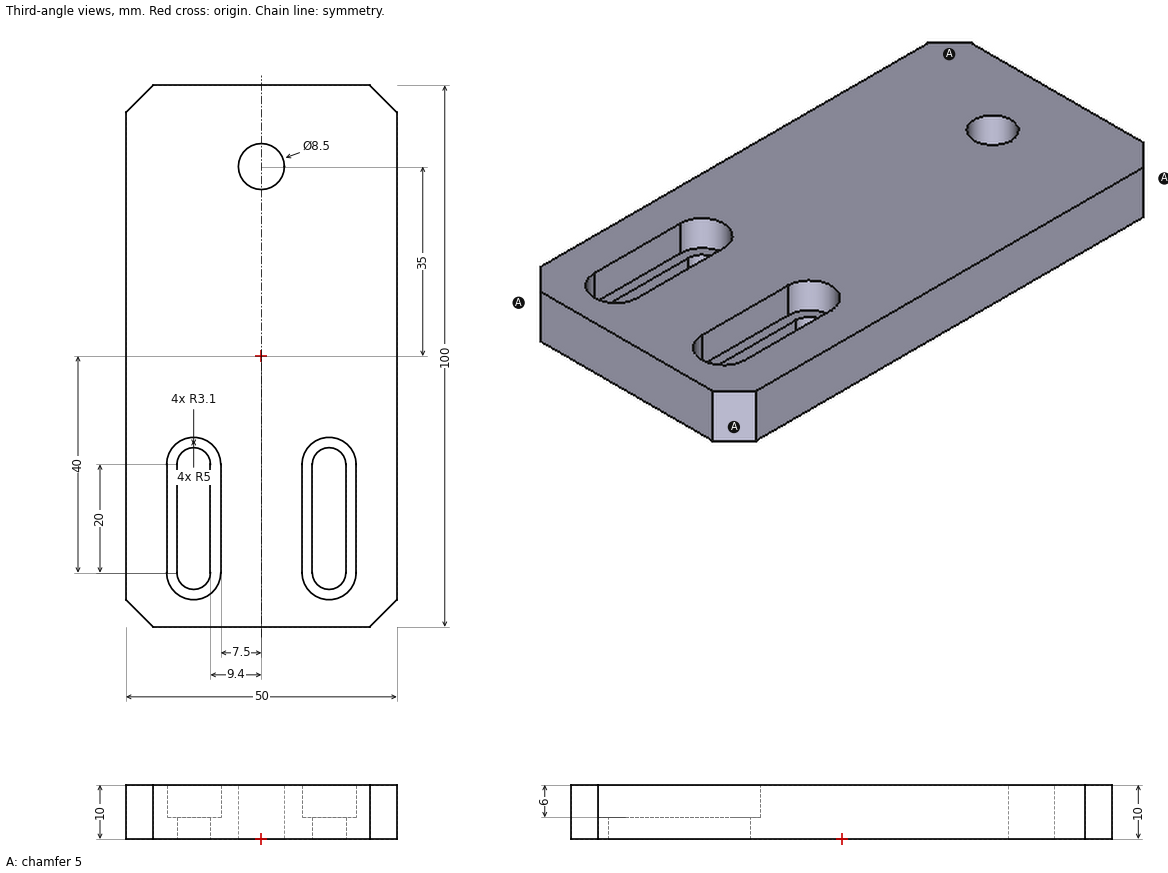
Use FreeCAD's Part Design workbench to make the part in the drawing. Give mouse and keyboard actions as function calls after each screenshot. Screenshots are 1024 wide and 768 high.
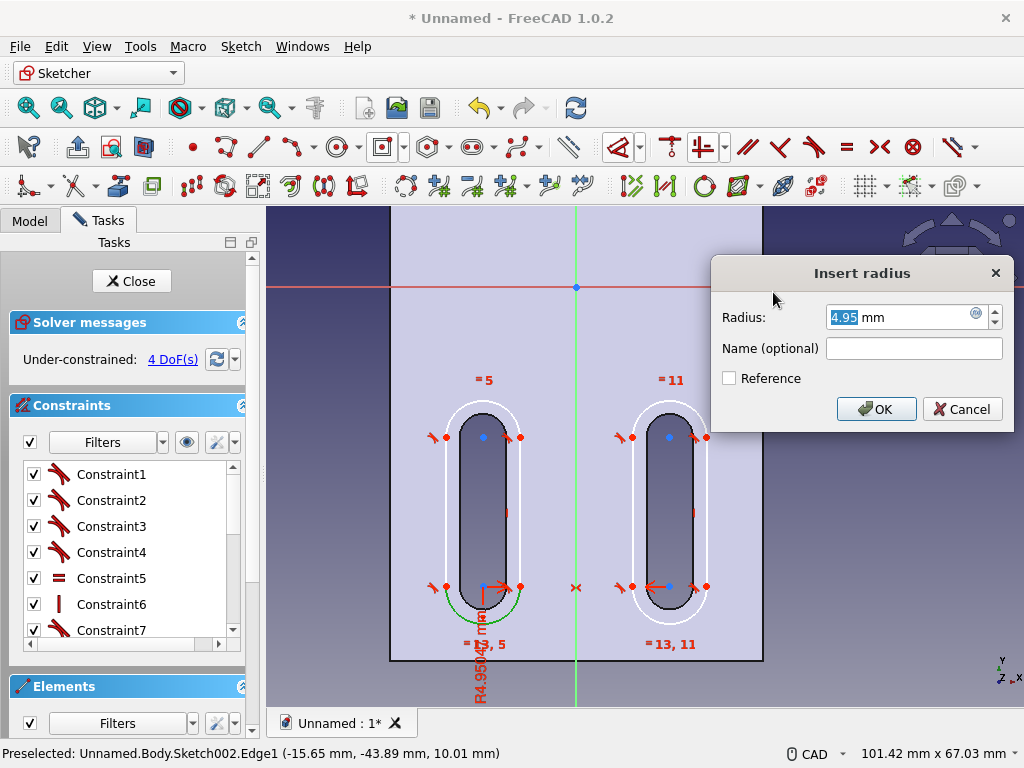
text(5)
key(Return)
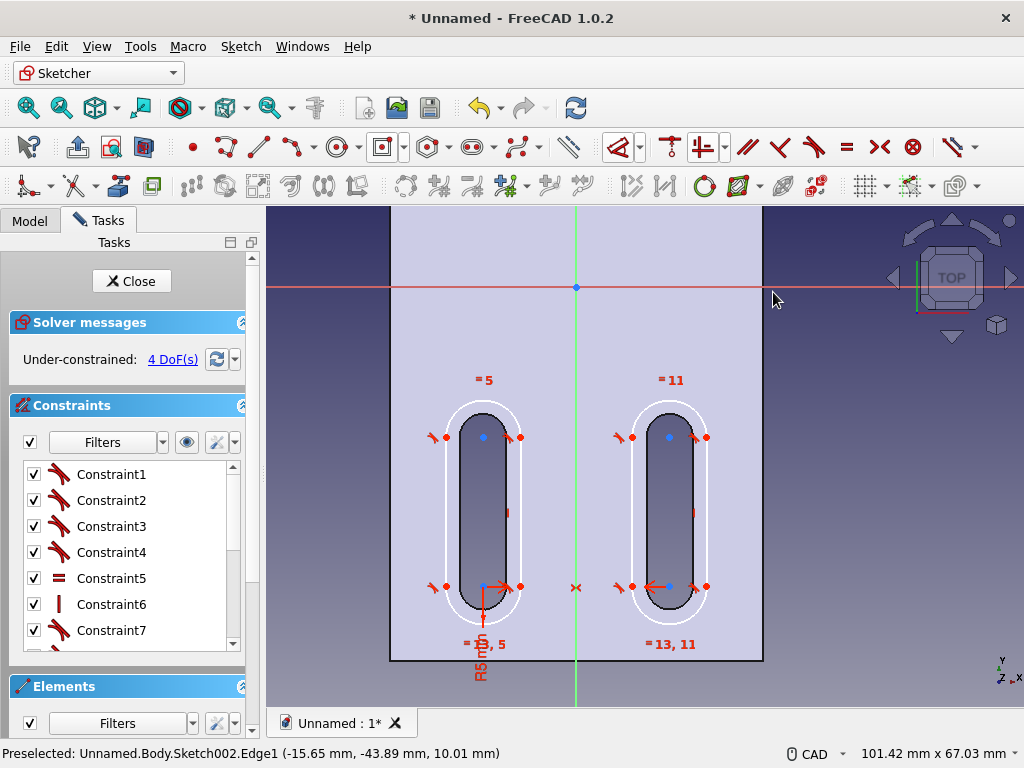
click(446, 542)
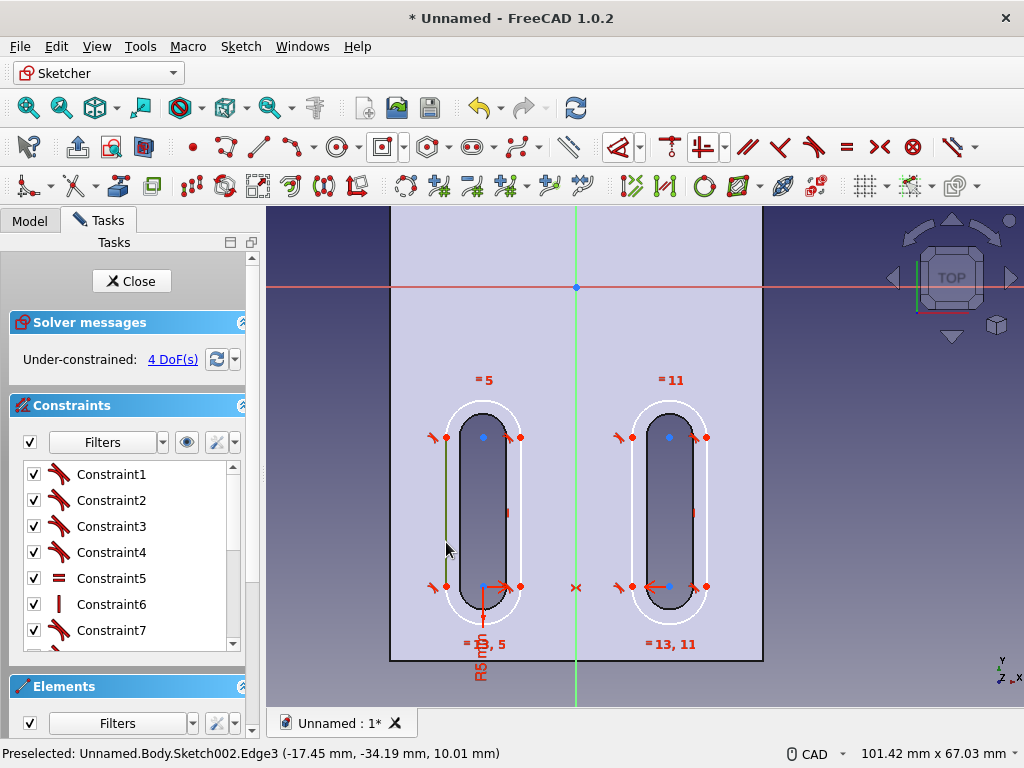
key(i)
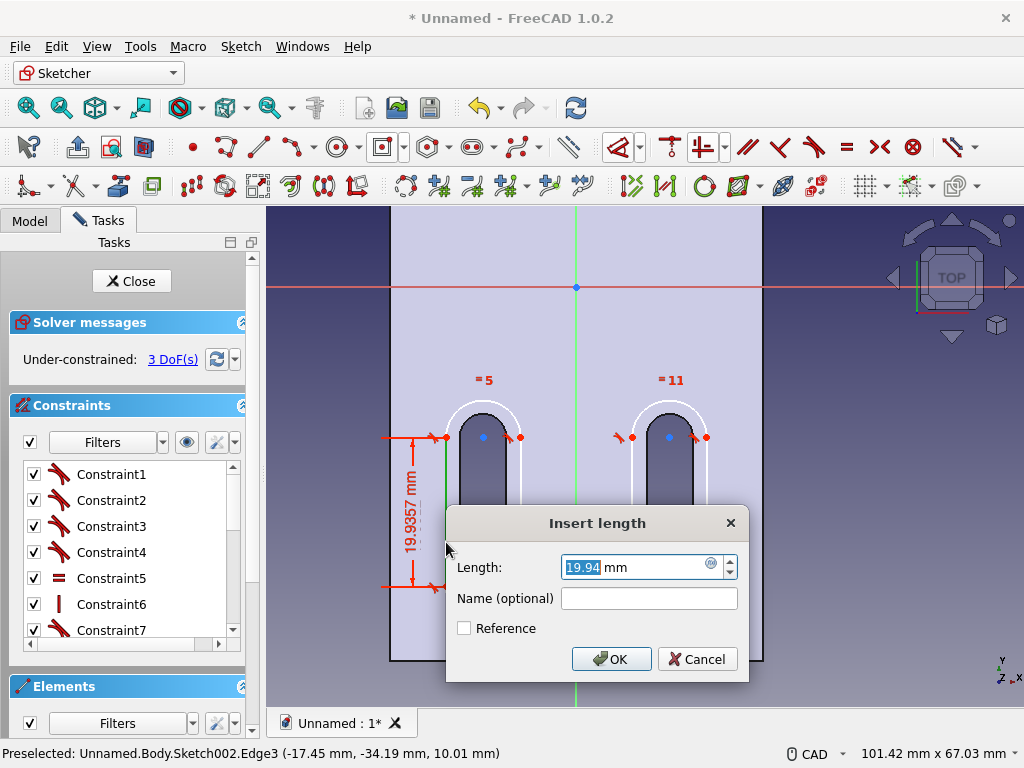
text(20)
key(Return)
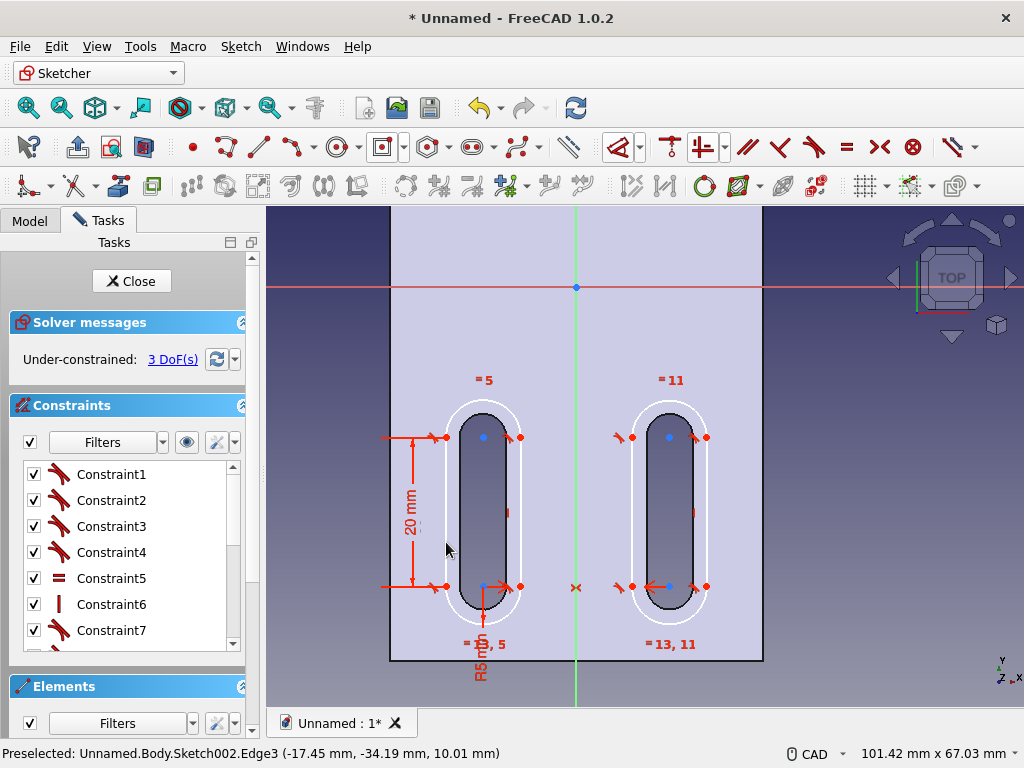
click(632, 542)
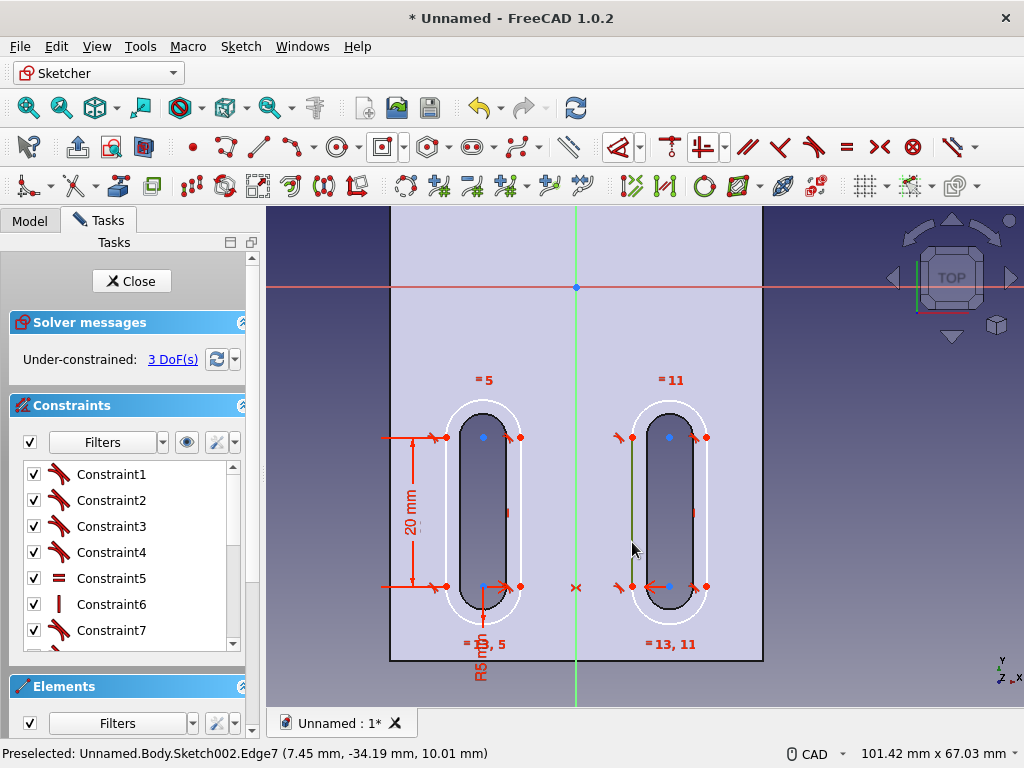
click(640, 148)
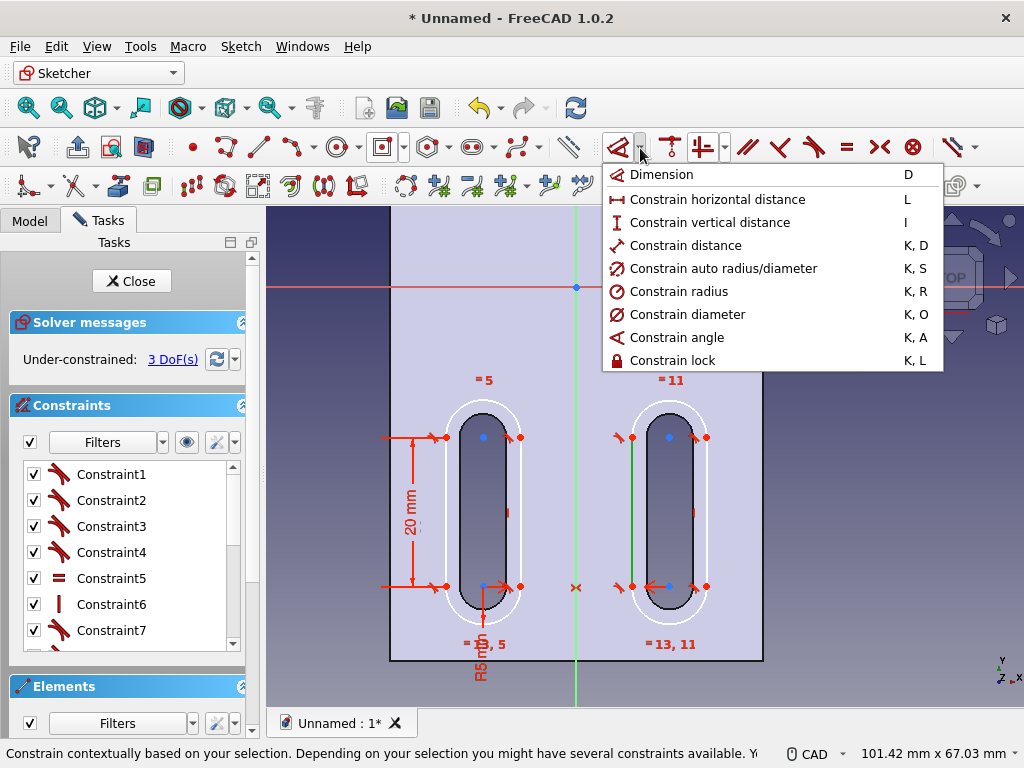
click(773, 222)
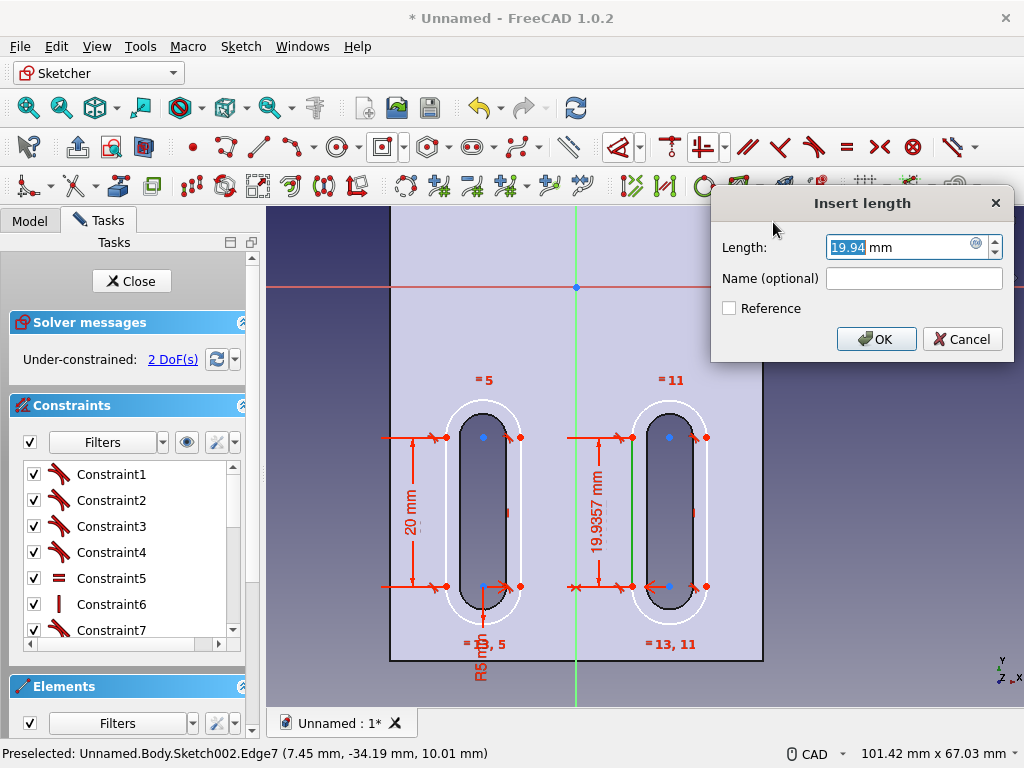
text(20)
key(Return)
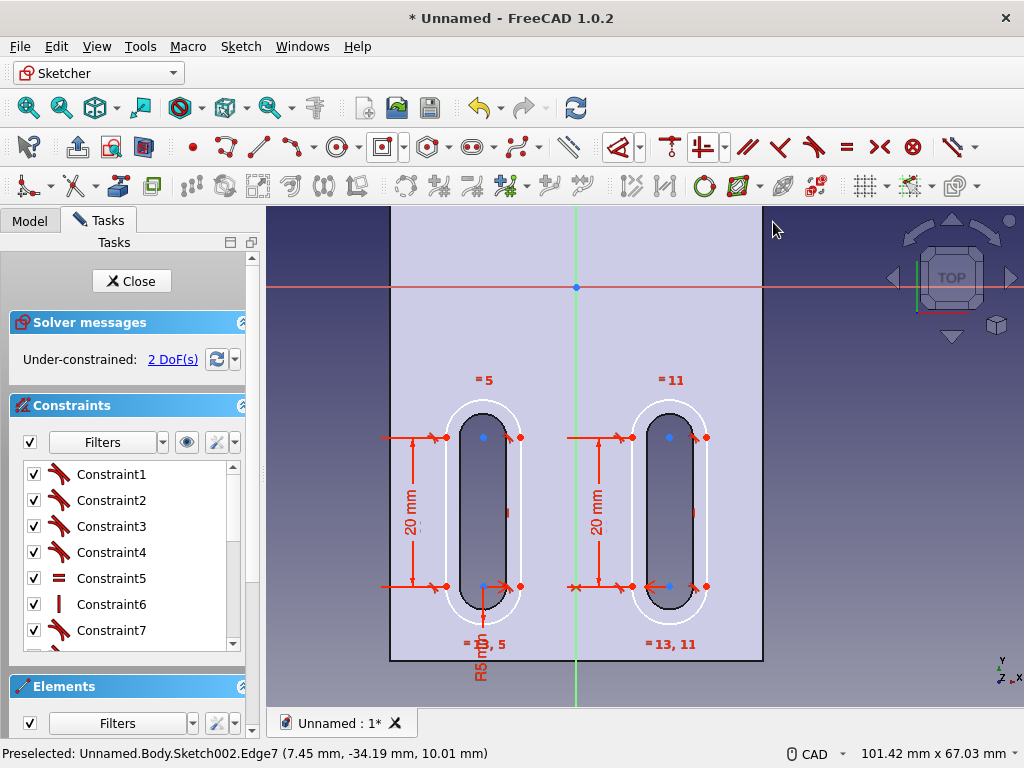
click(446, 587)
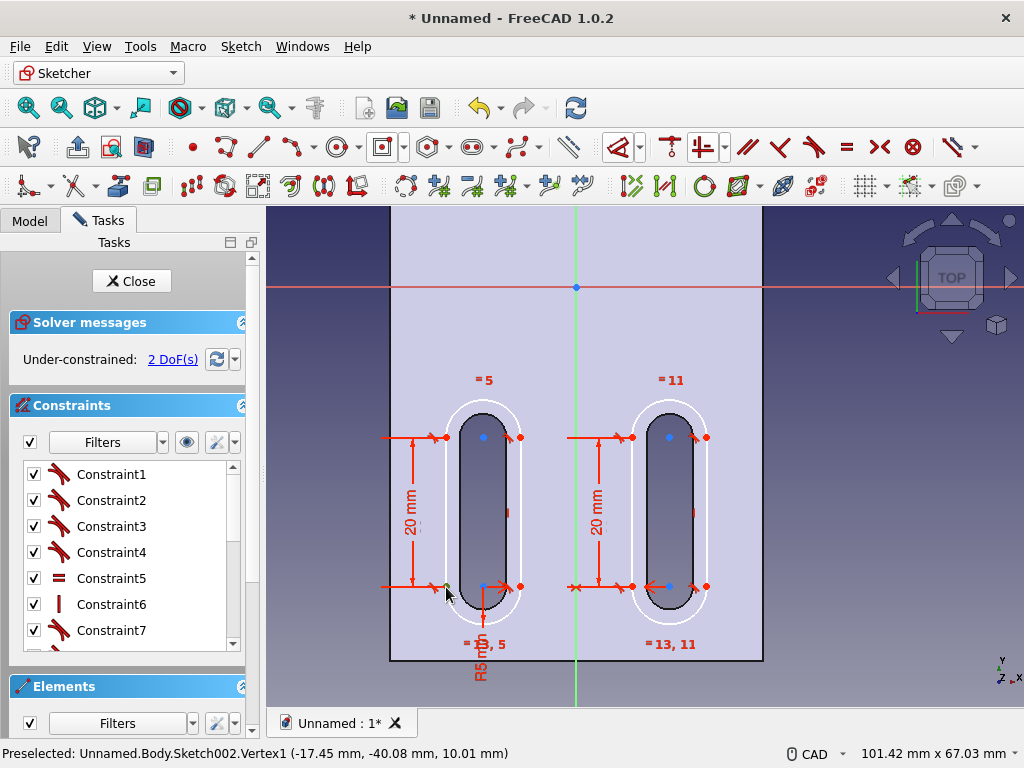
key(i)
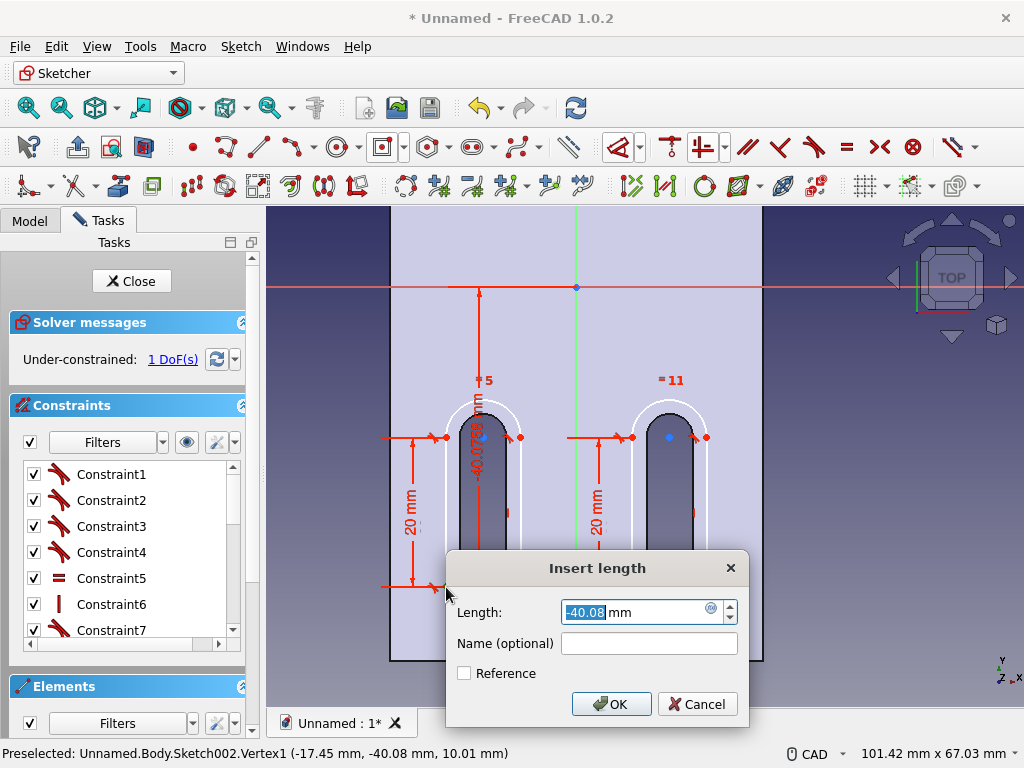
text(-40)
key(Return)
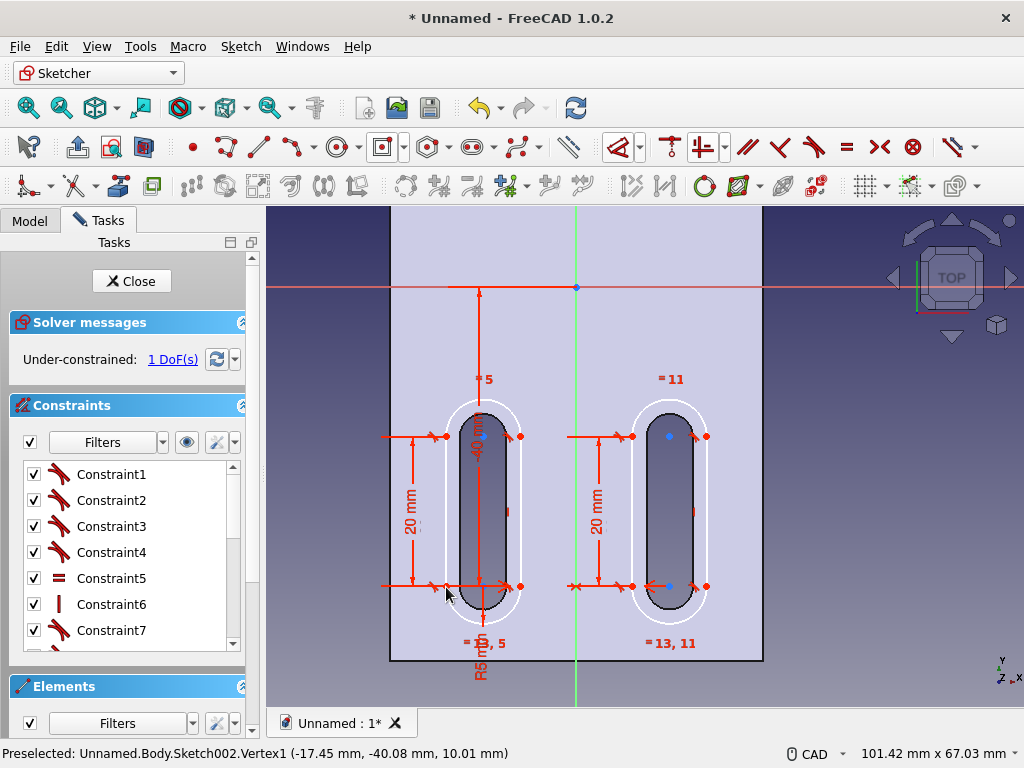
click(521, 586)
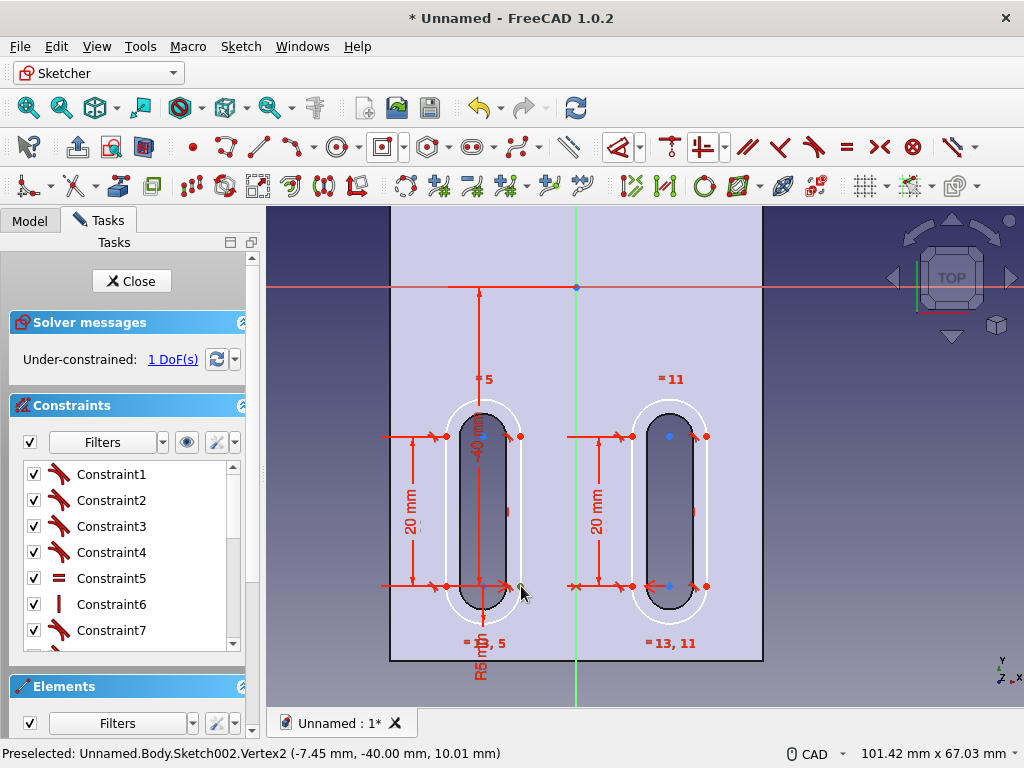
click(640, 148)